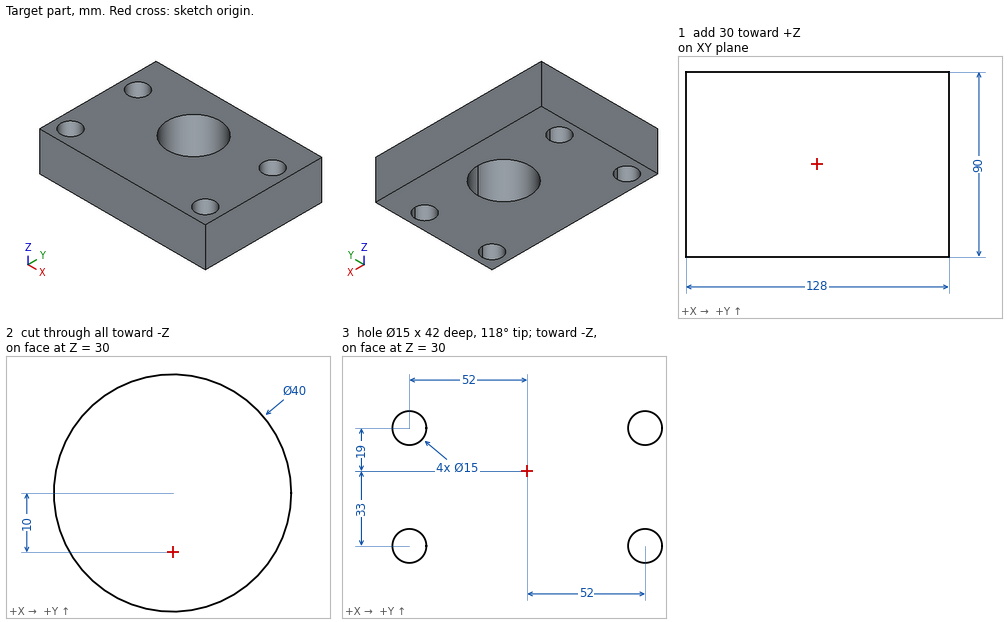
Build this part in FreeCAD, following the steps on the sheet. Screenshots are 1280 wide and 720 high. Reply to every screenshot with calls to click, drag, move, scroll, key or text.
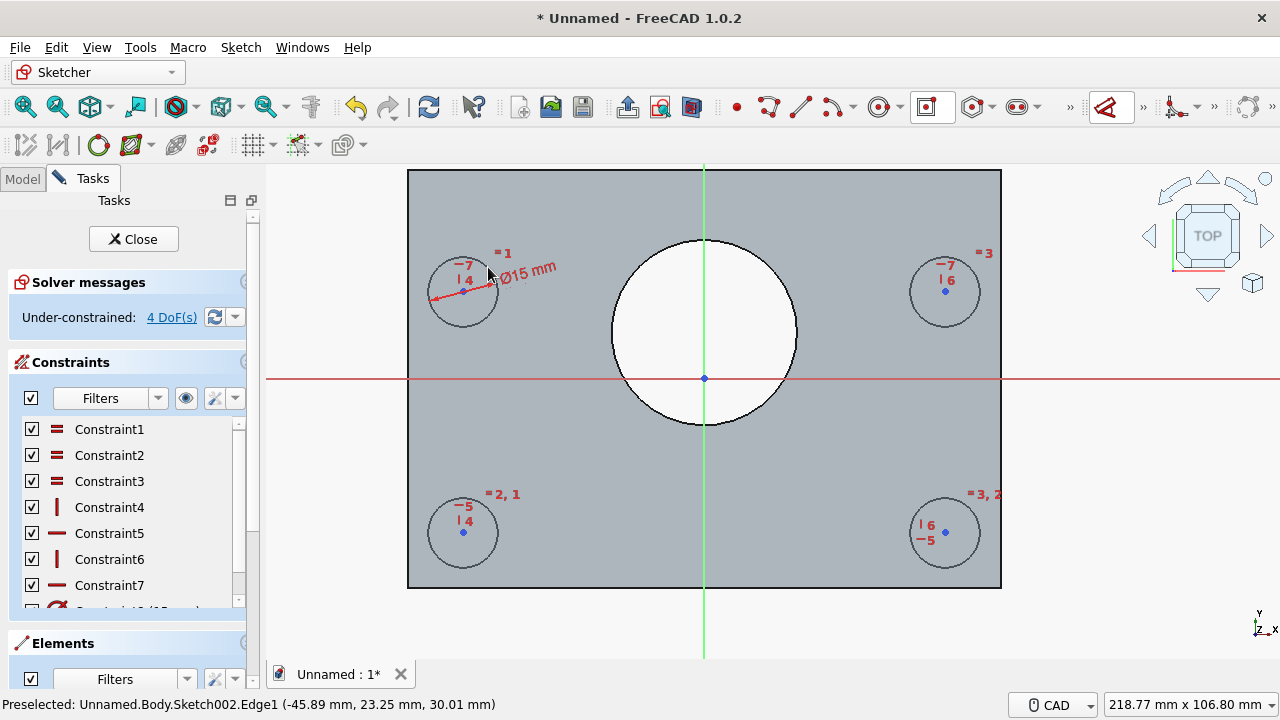
click(463, 292)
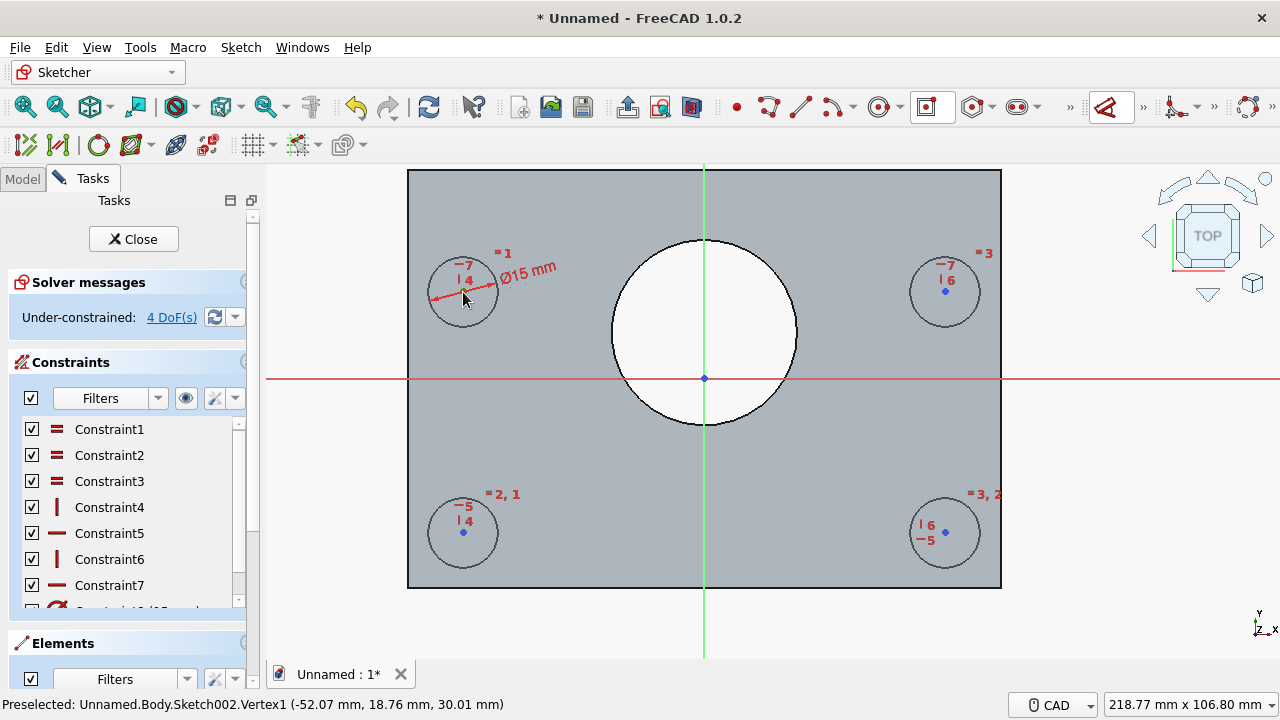
click(1128, 108)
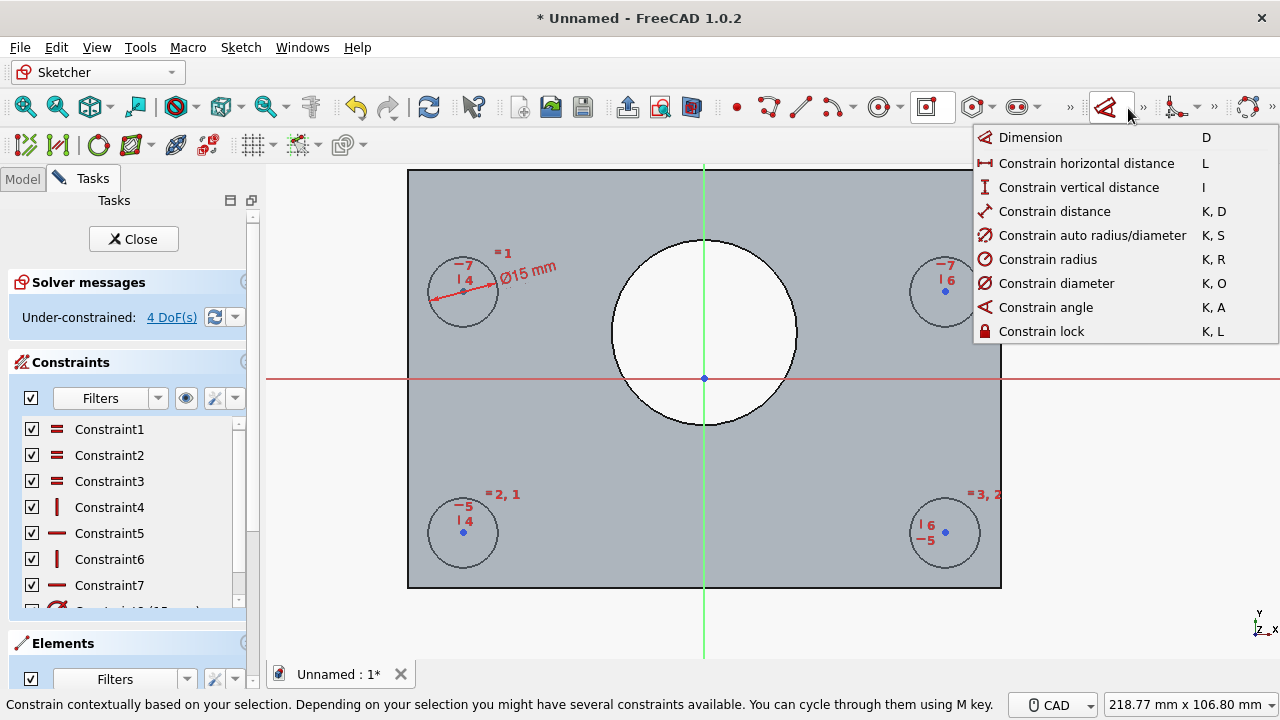
click(1126, 163)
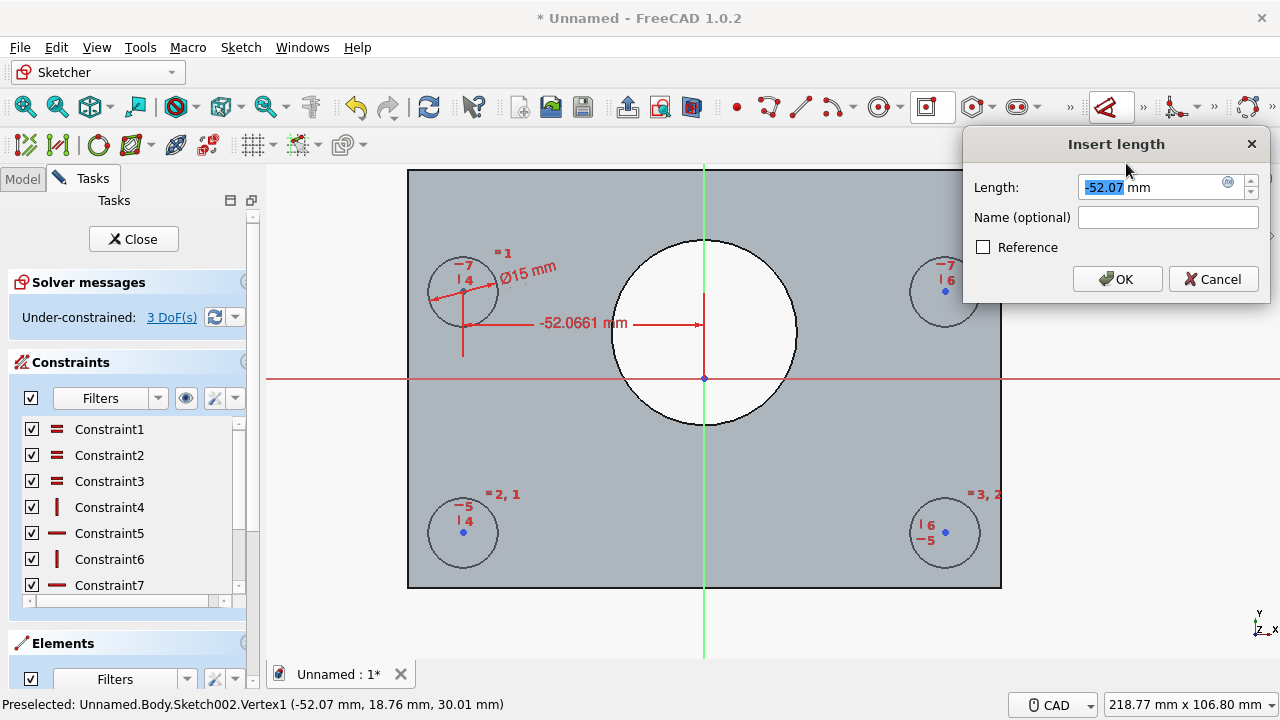
text(-52)
key(Return)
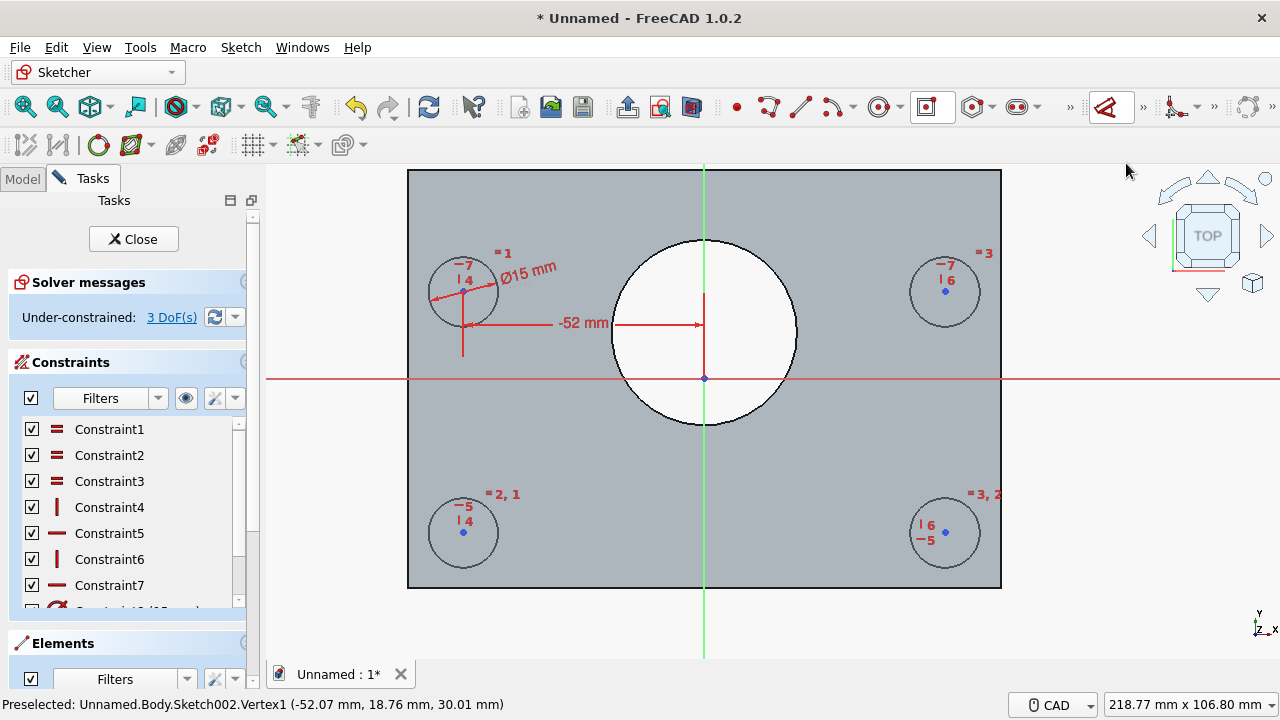
click(463, 292)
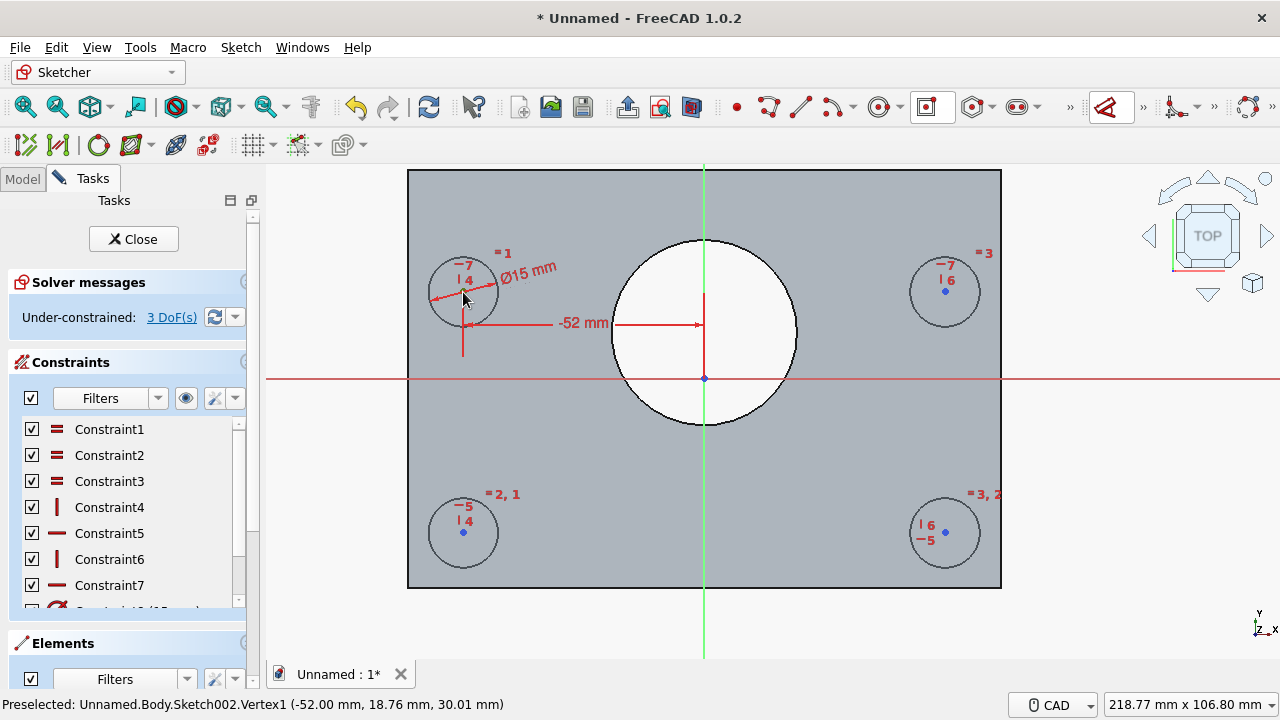
click(1128, 108)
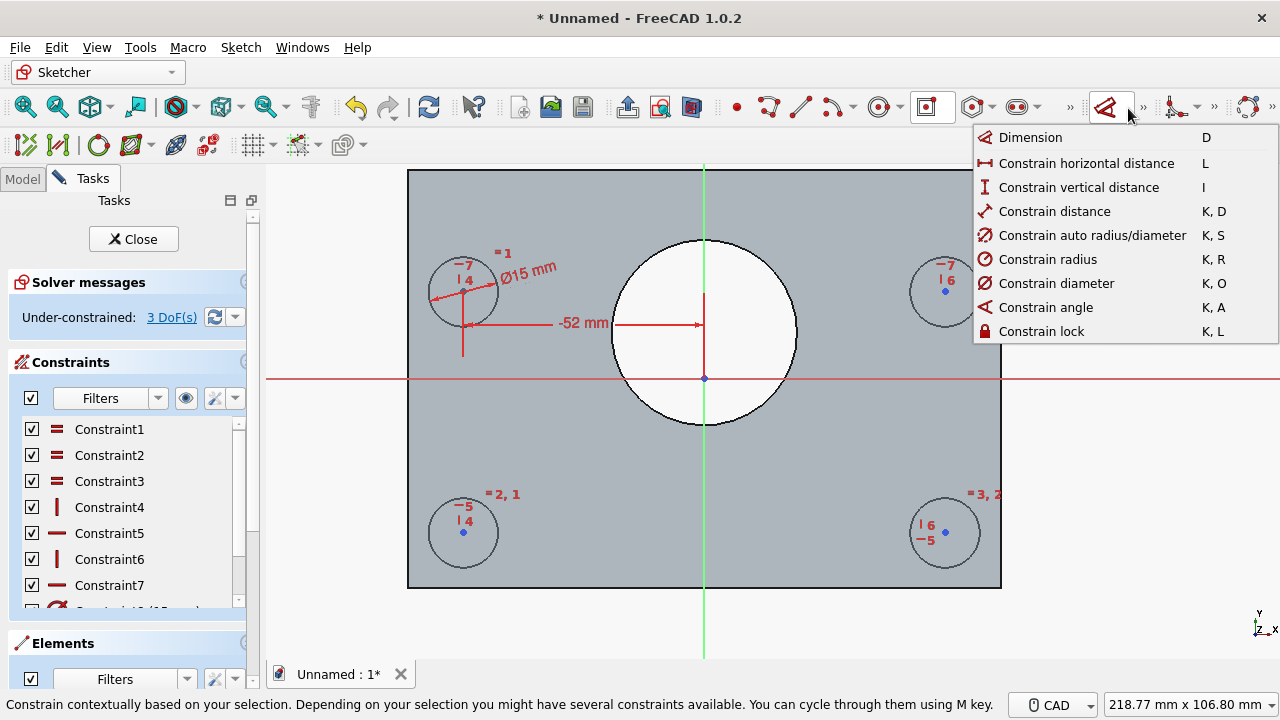
click(1126, 187)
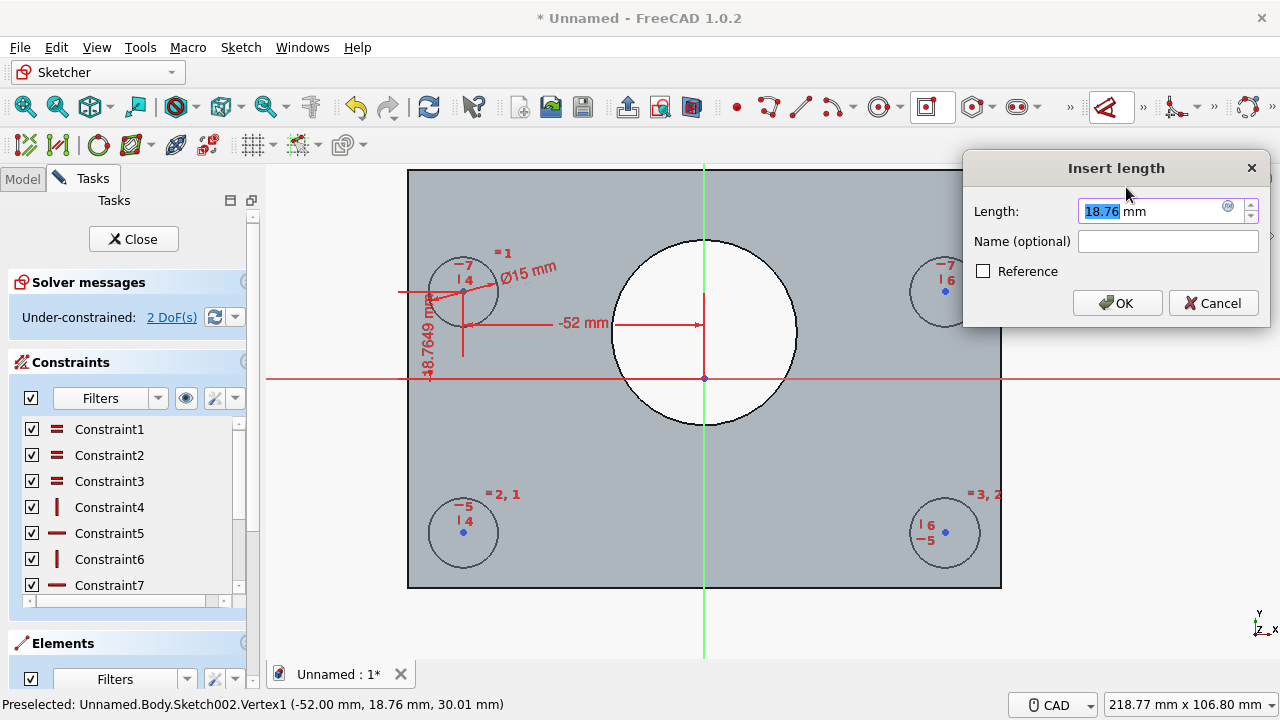
text(19)
key(Return)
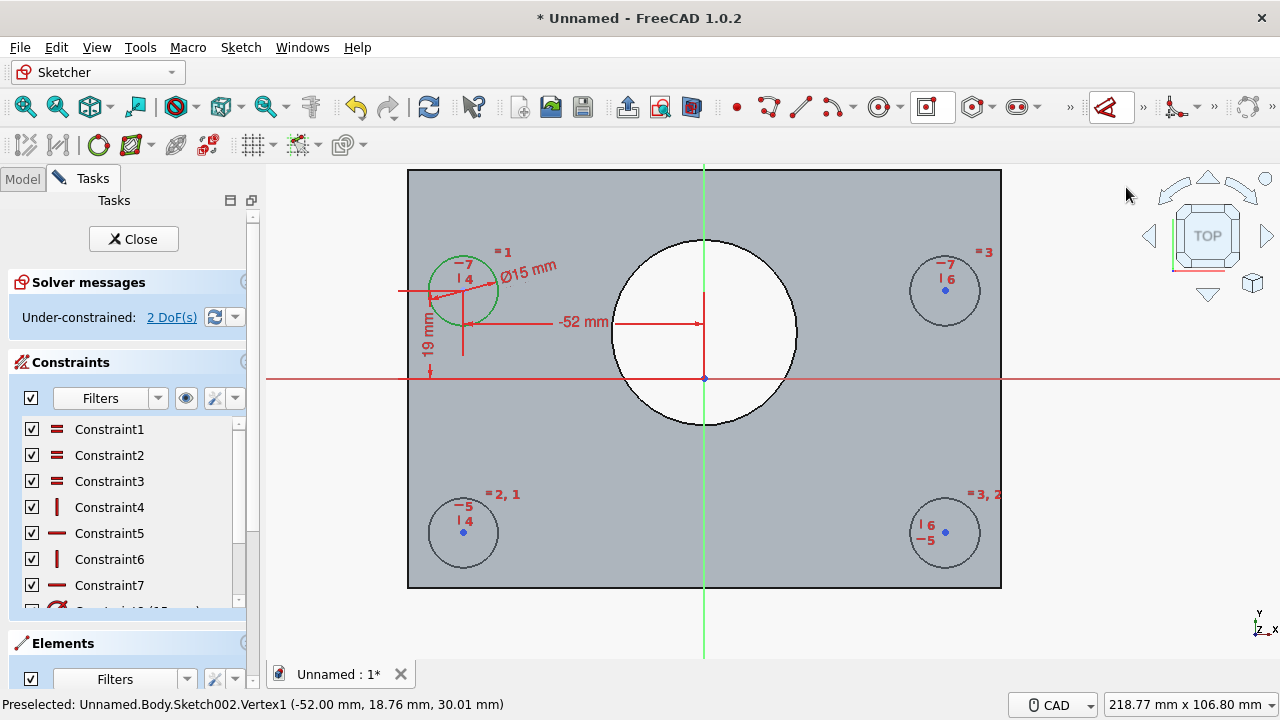
click(463, 533)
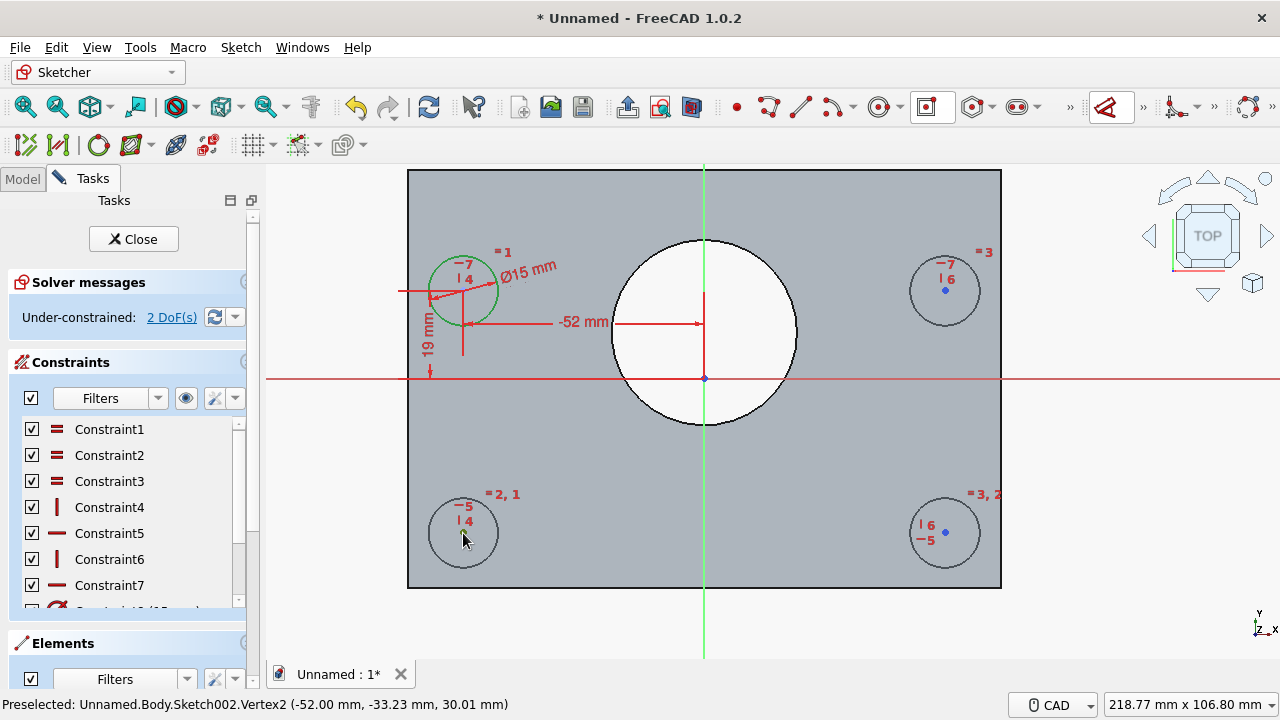
click(1128, 108)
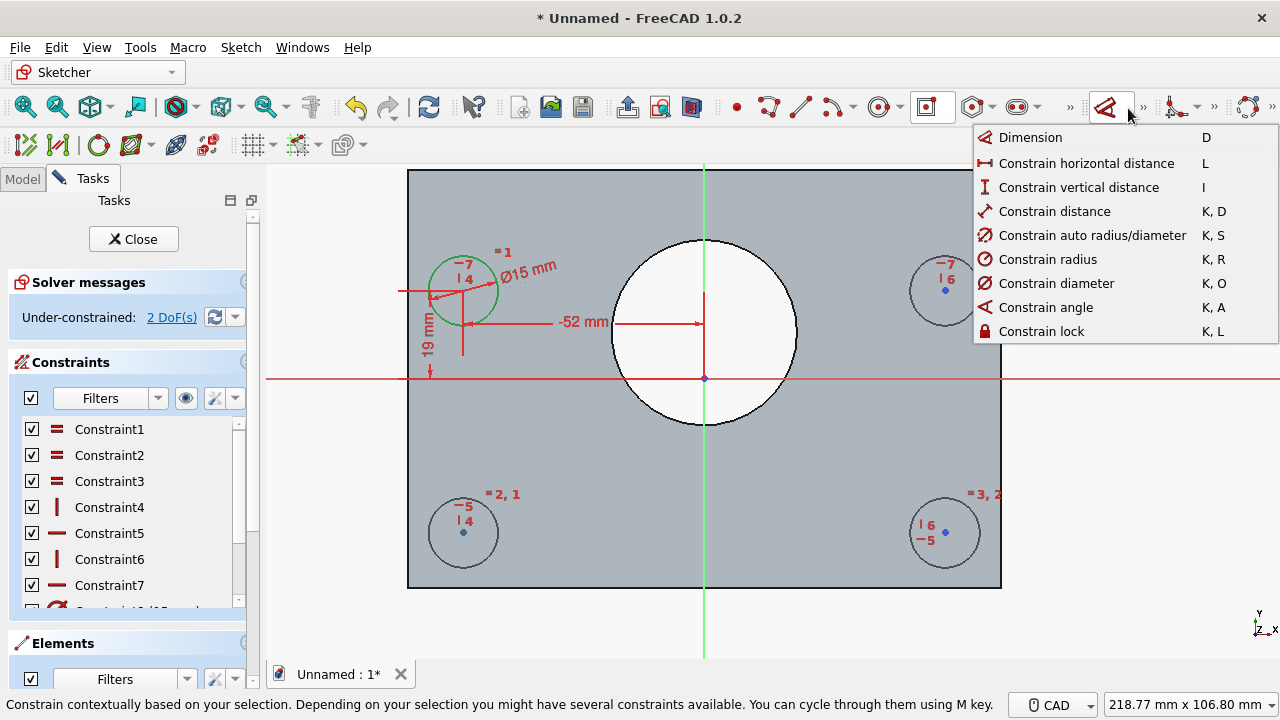
click(1126, 187)